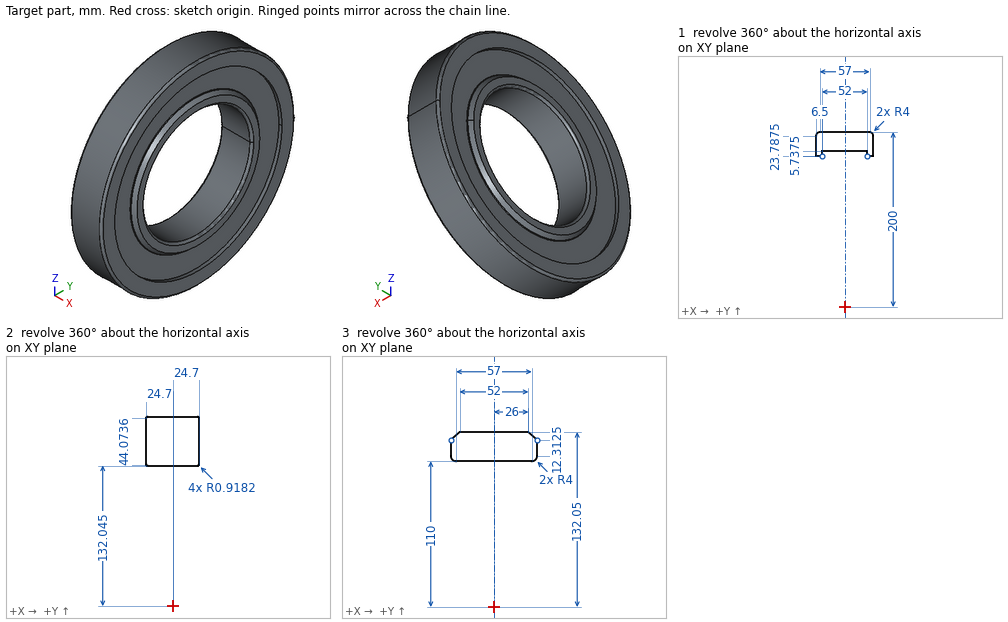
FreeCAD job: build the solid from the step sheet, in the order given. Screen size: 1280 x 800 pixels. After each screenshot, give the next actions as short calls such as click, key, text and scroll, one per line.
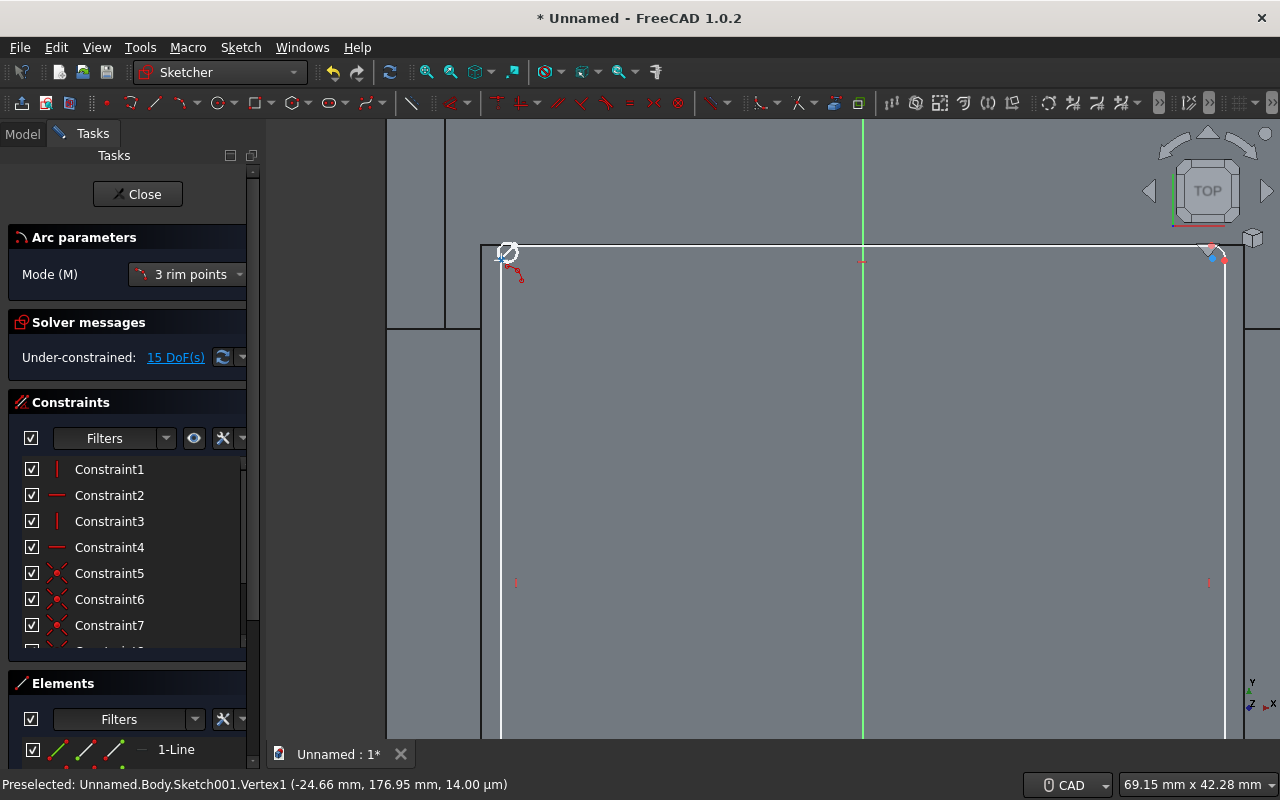
scroll(504, 249, up, 7)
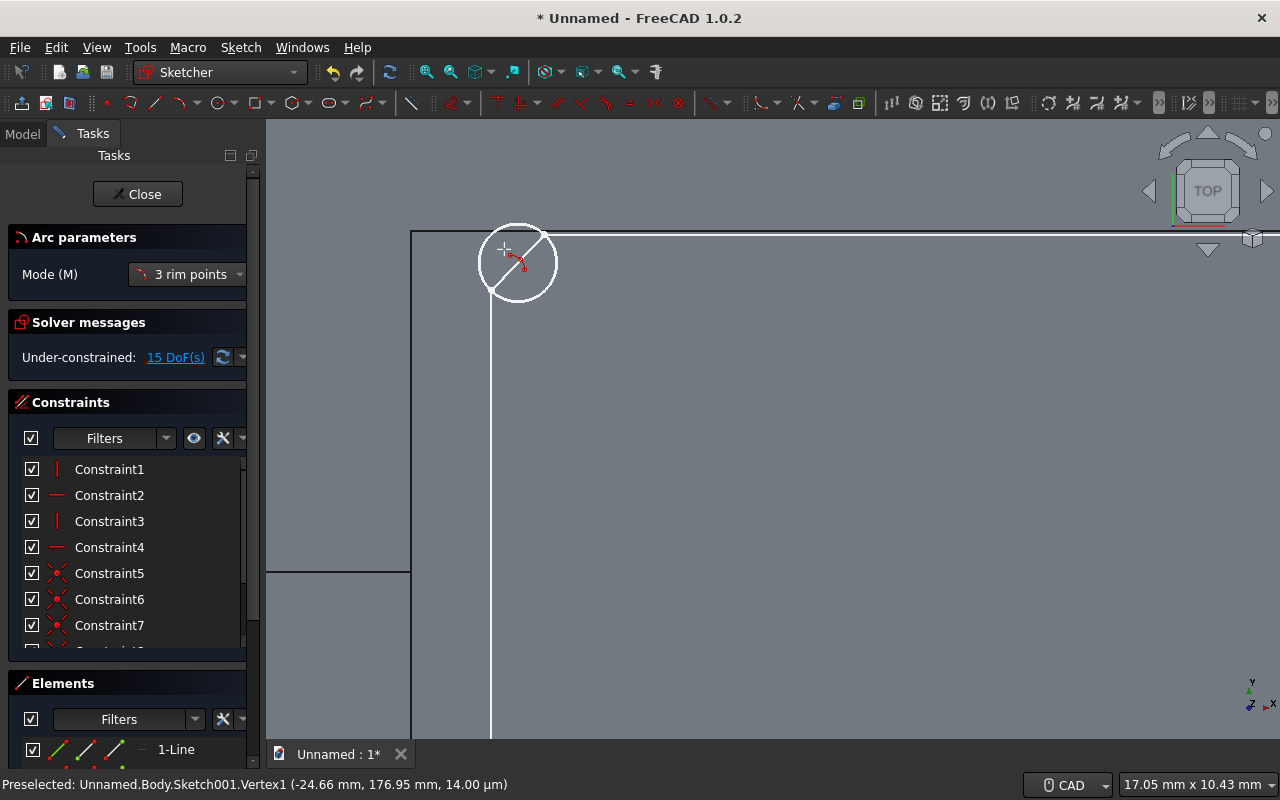
click(505, 247)
key(Escape)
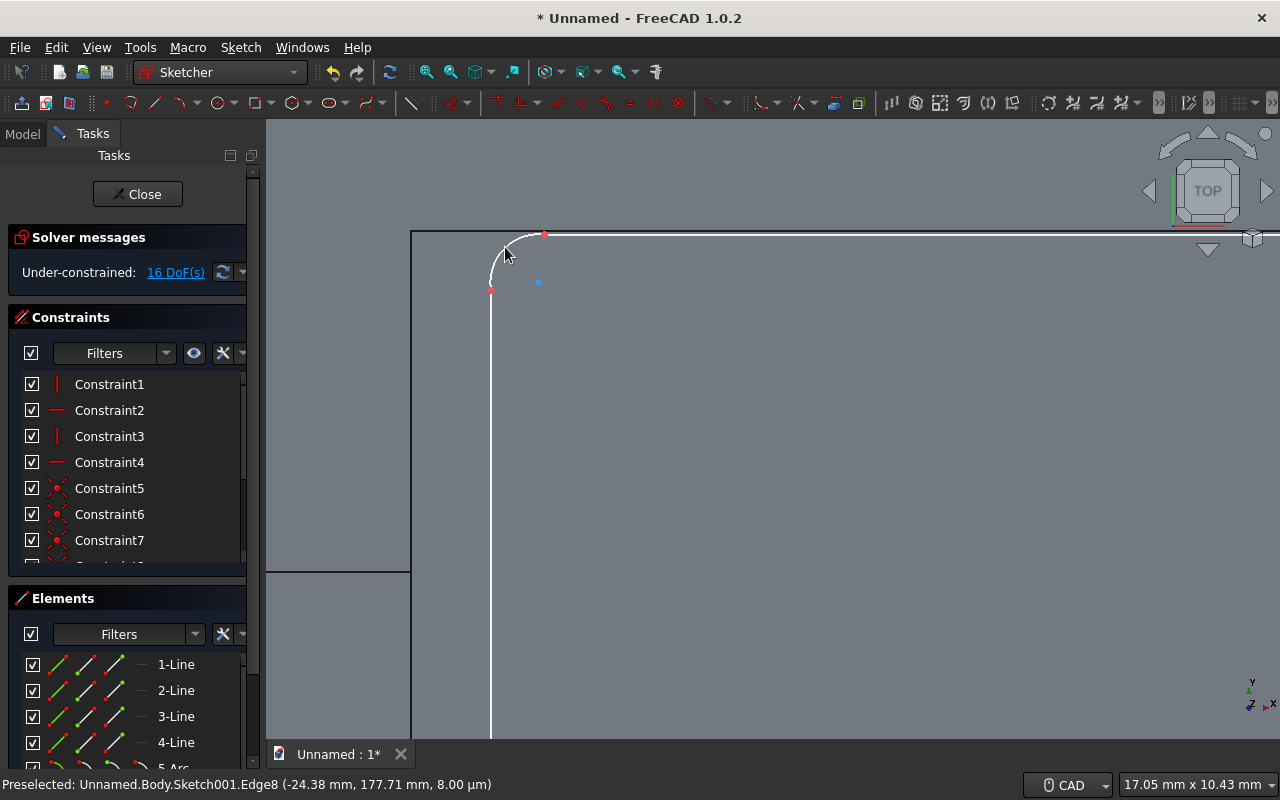
scroll(508, 246, down, 10)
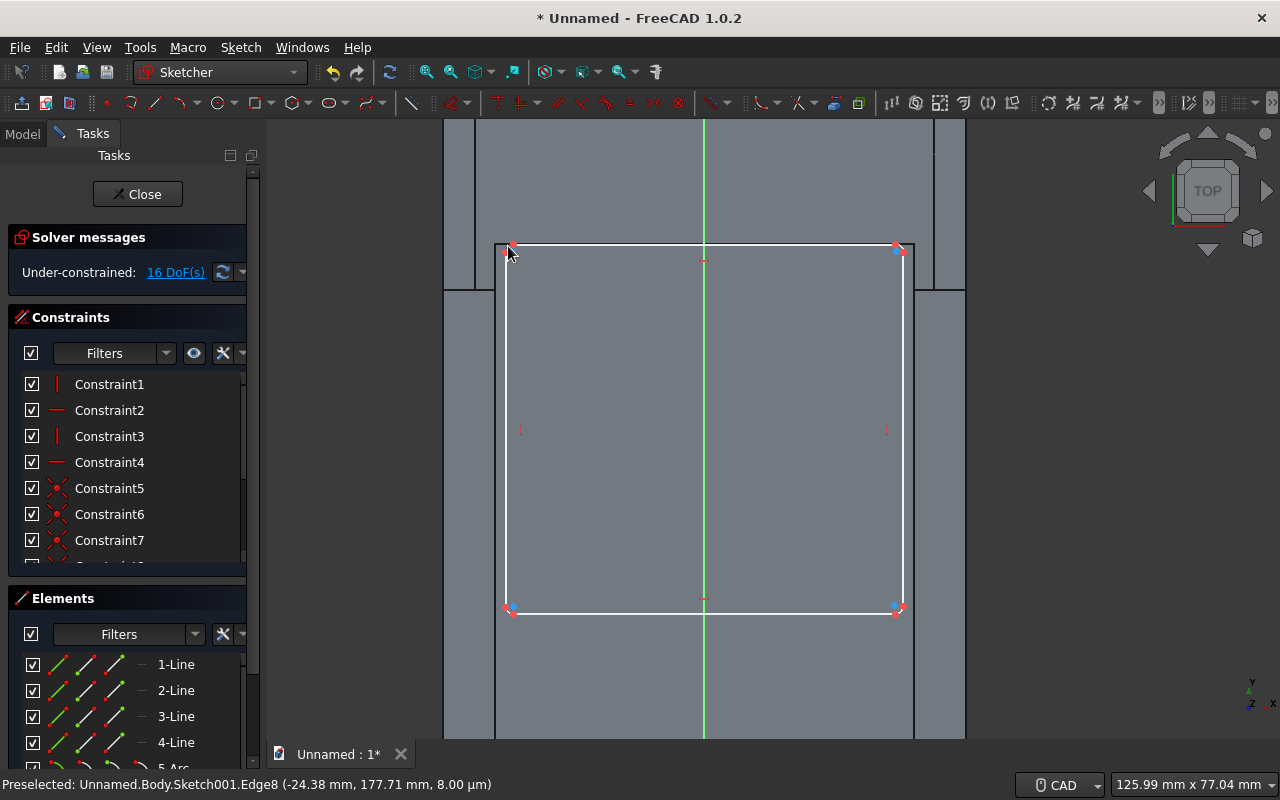
click(506, 359)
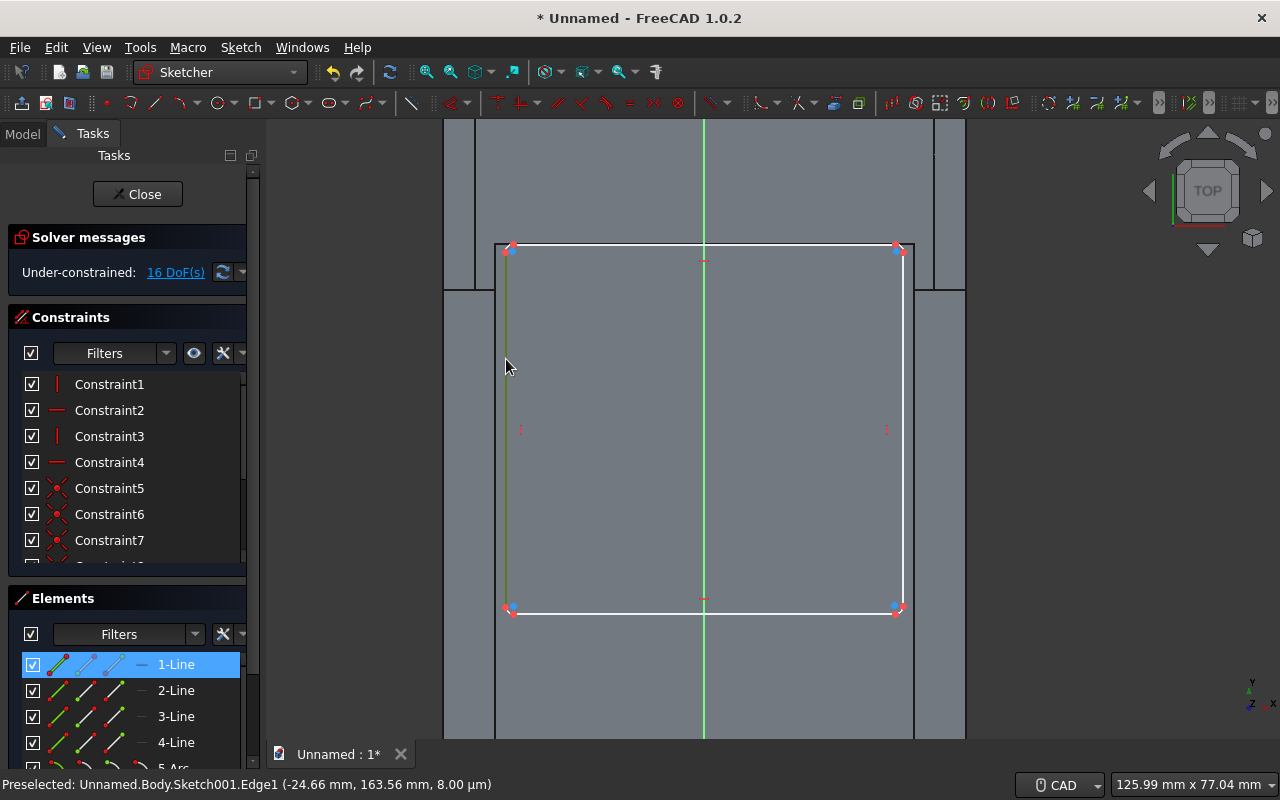
scroll(508, 612, up, 5)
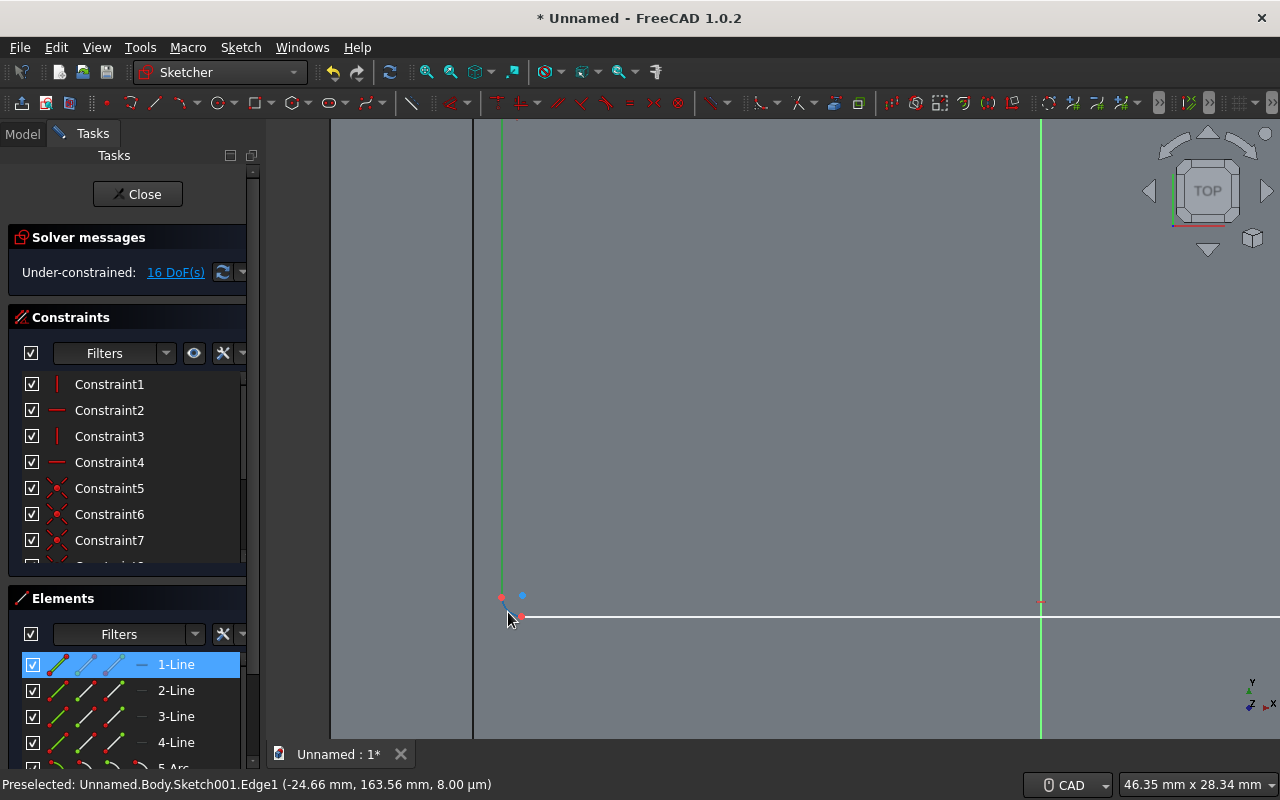
click(508, 611)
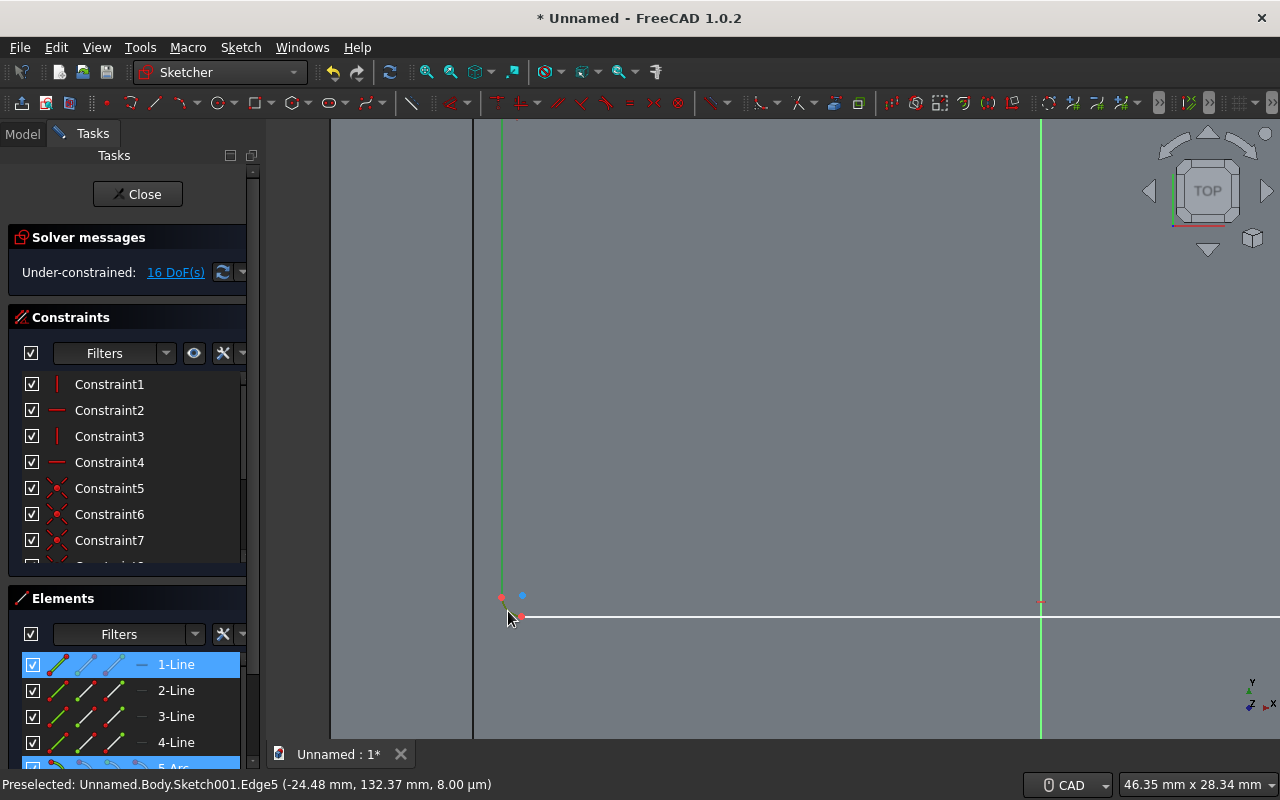
click(606, 104)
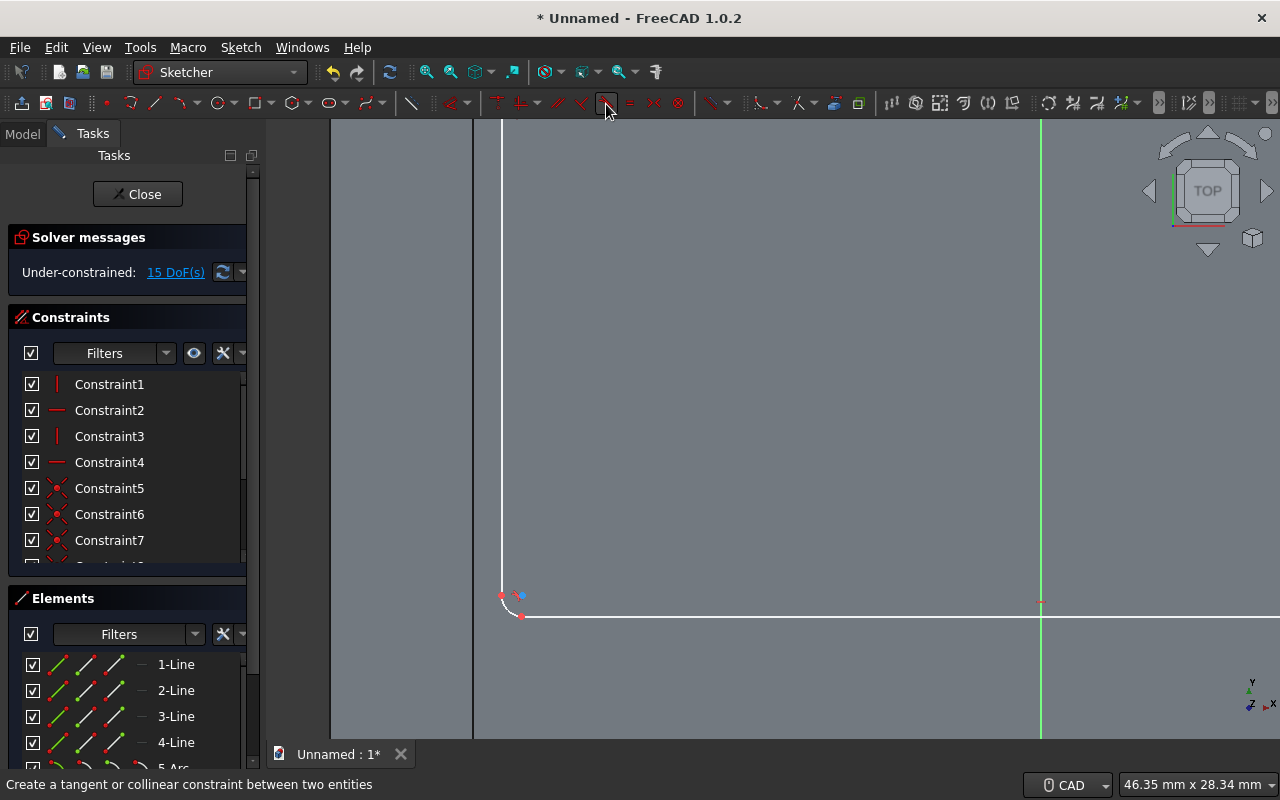
click(502, 307)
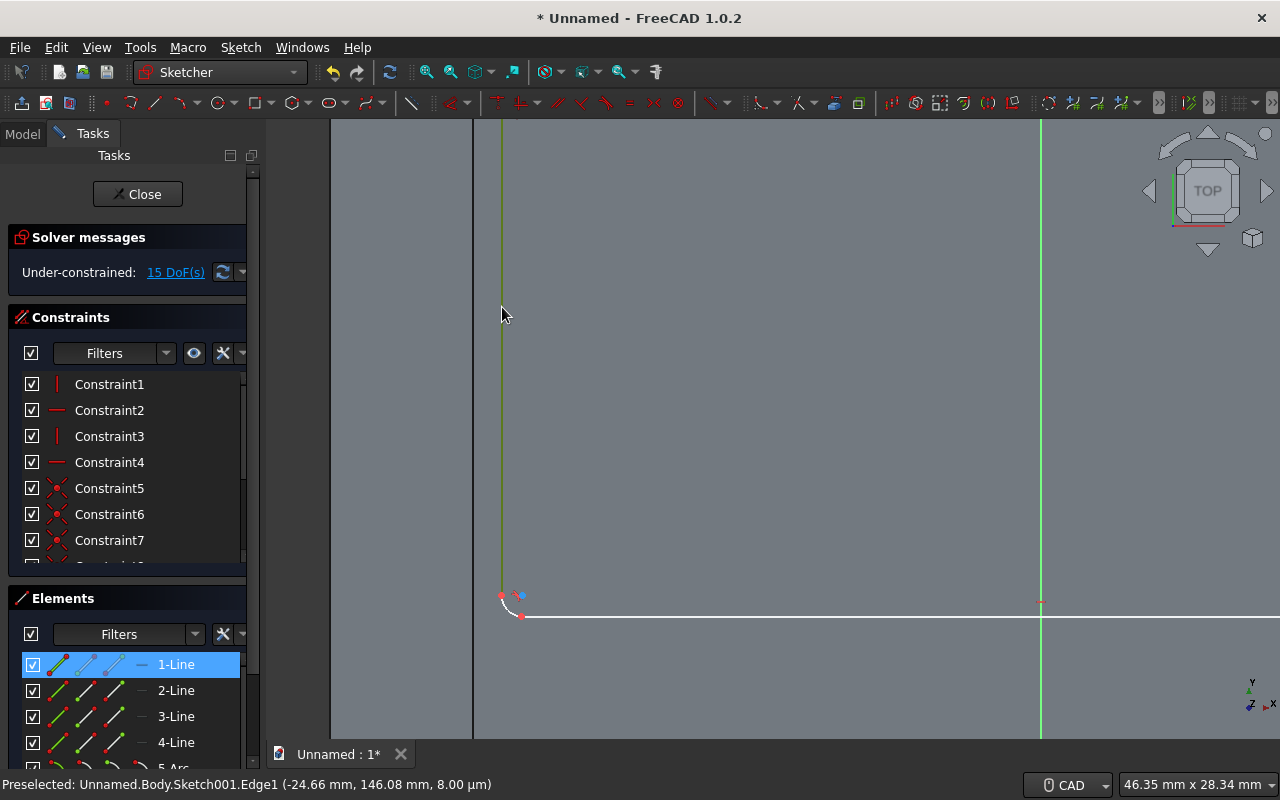
scroll(508, 613, down, 5)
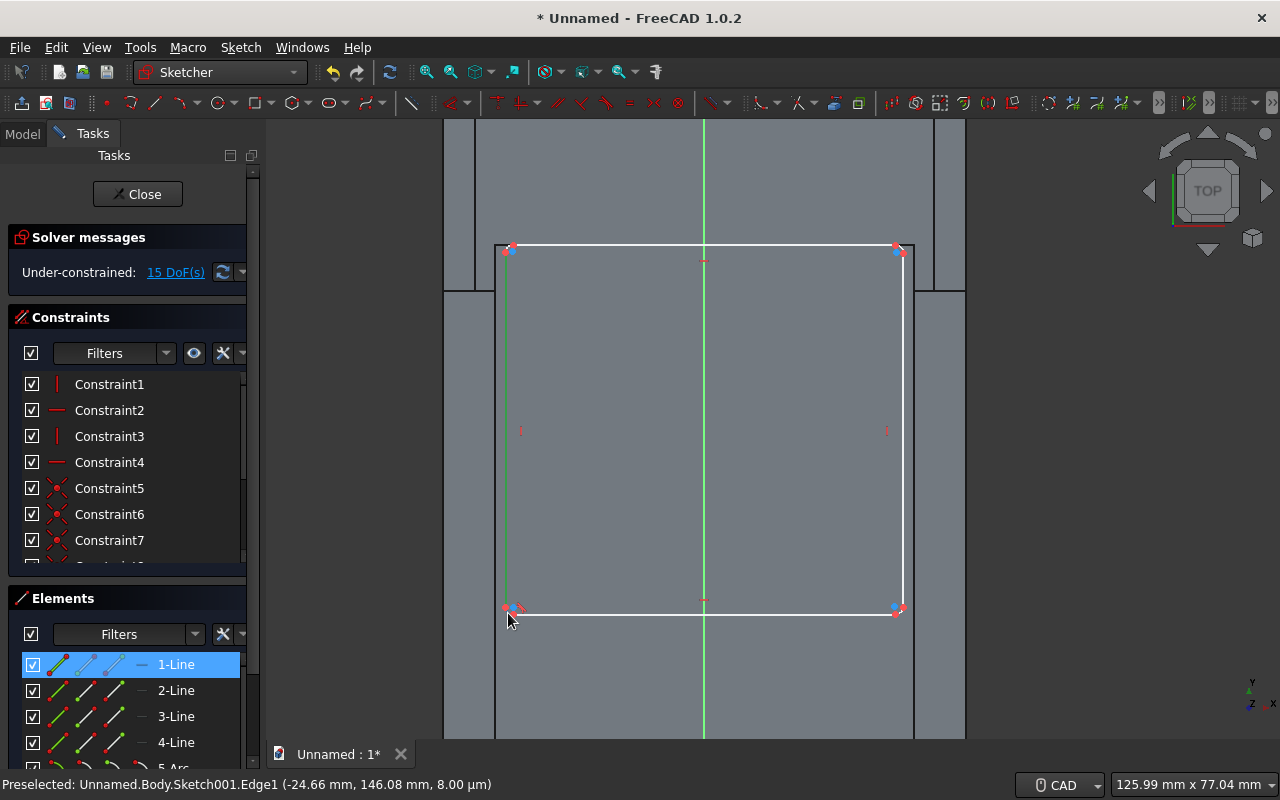
scroll(510, 246, up, 7)